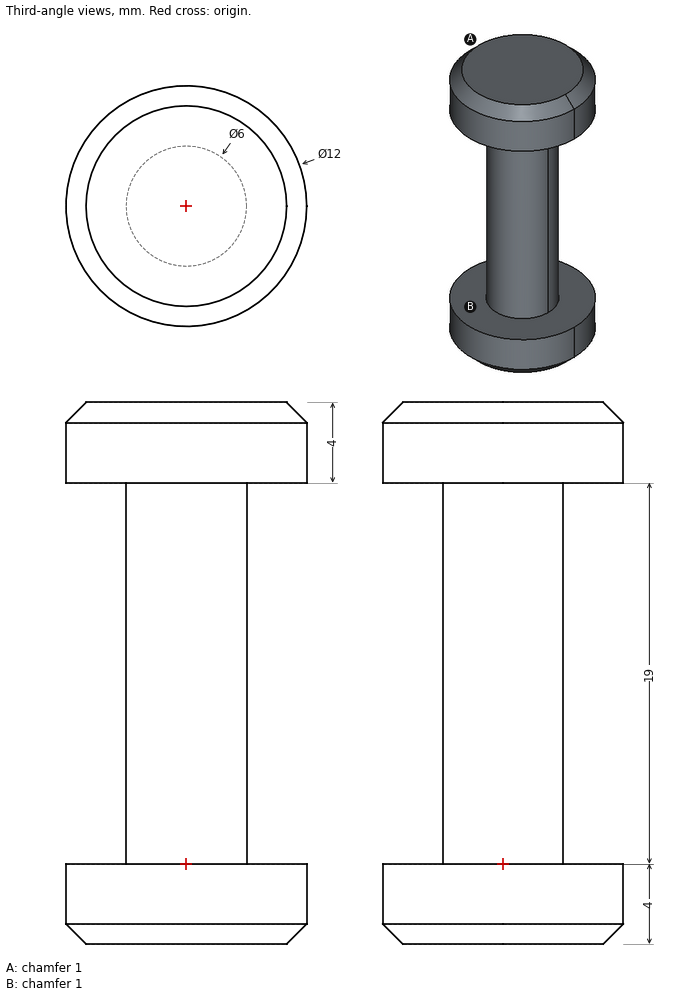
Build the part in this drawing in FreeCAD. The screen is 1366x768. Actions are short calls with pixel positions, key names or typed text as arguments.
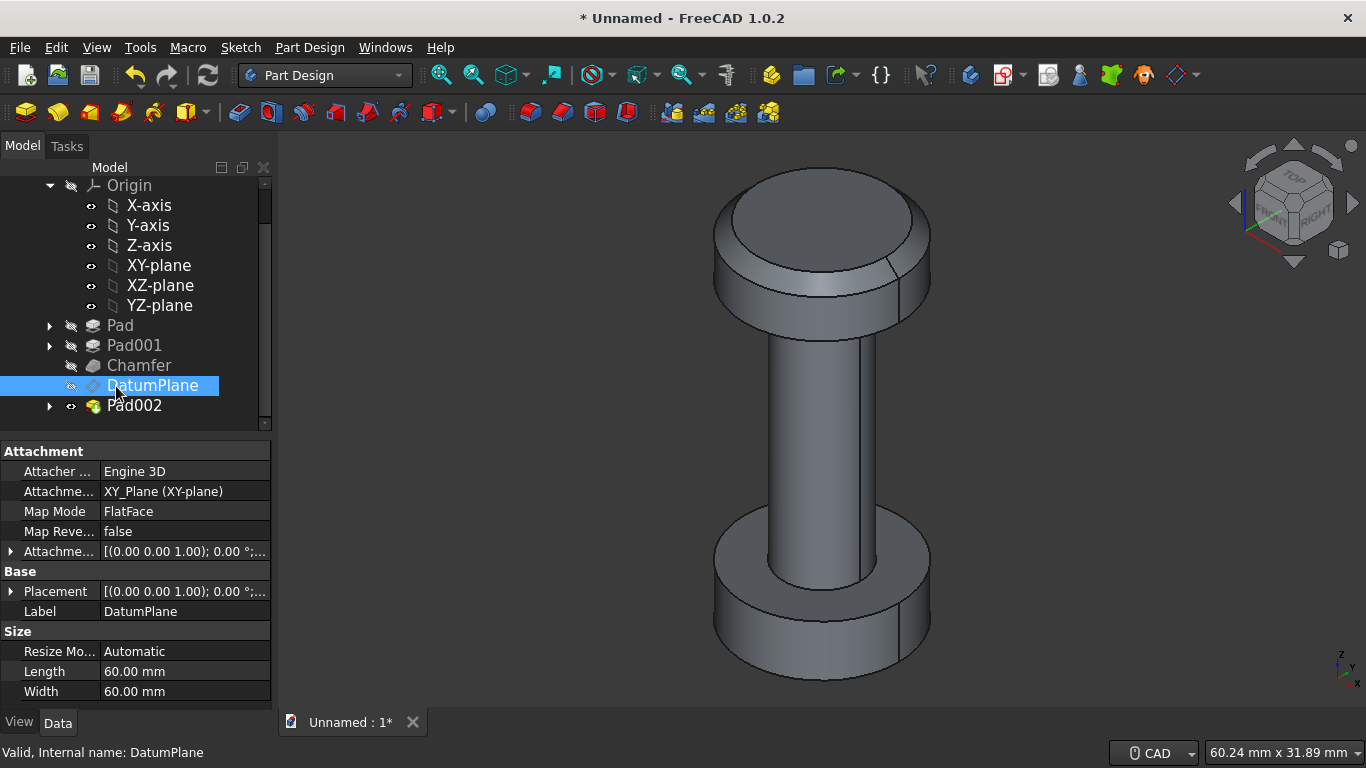
key(v)
key(f)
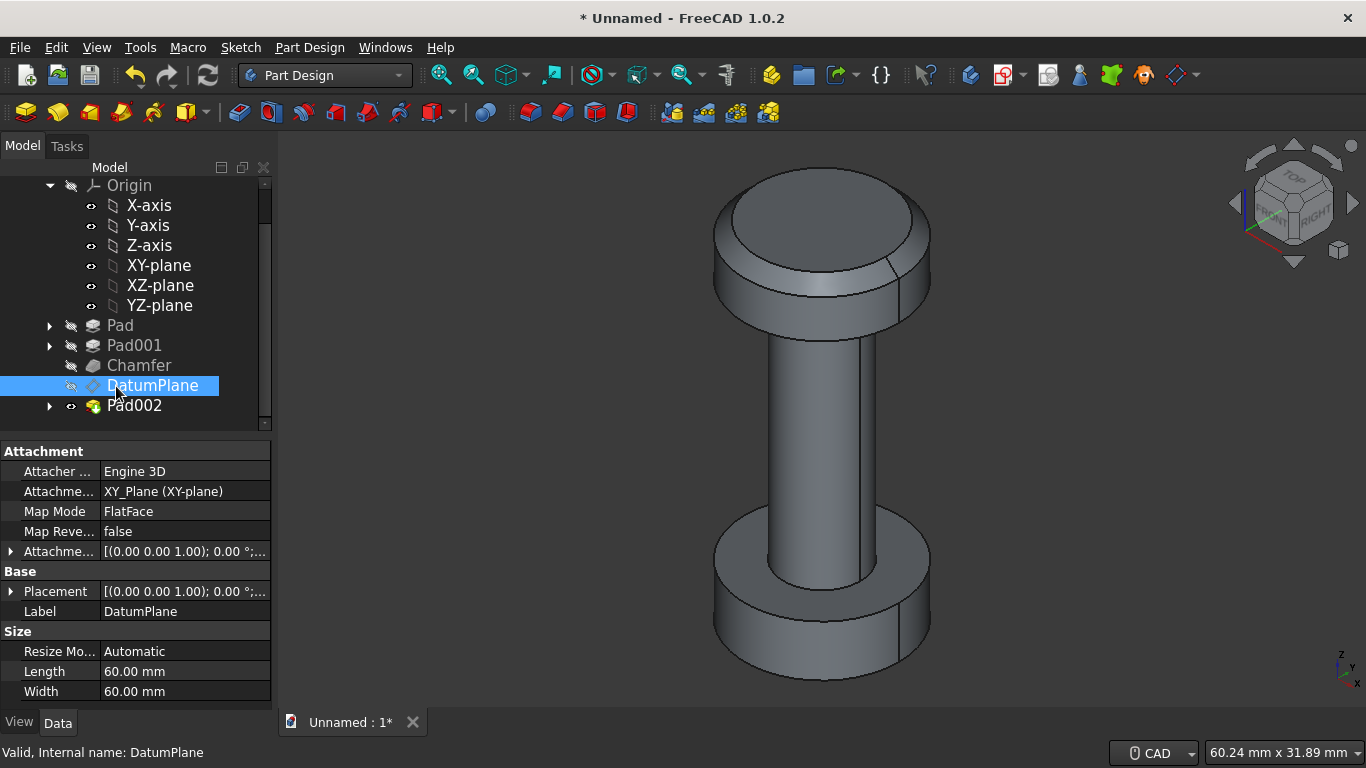
click(912, 652)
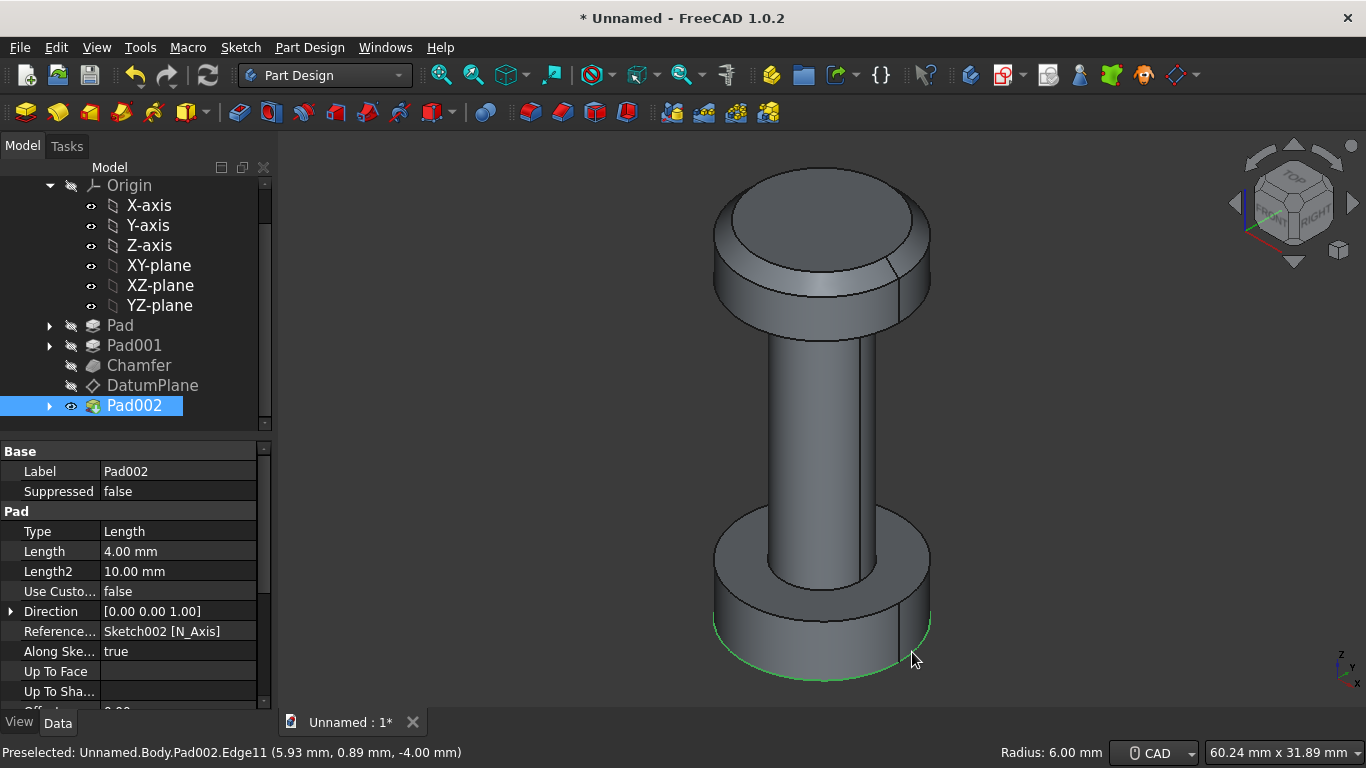
click(564, 112)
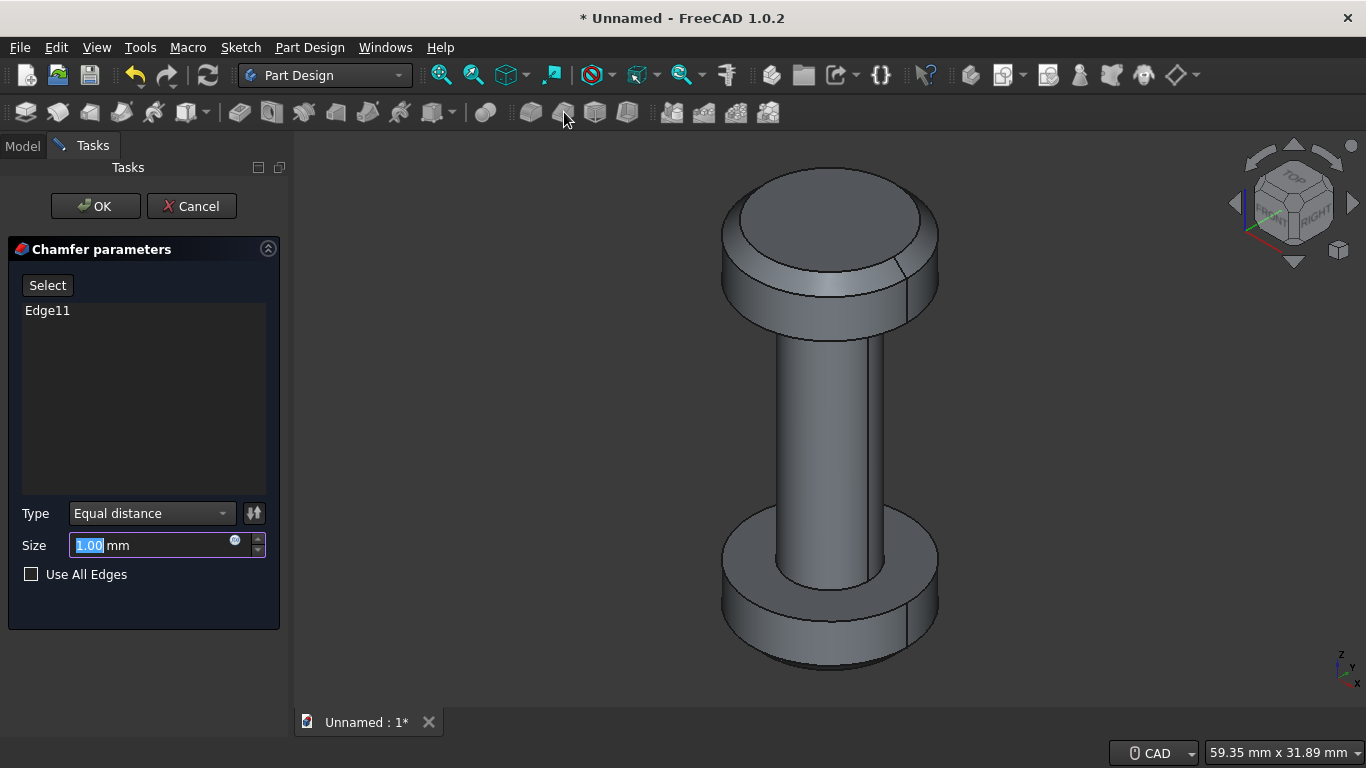
text(1)
key(Tab)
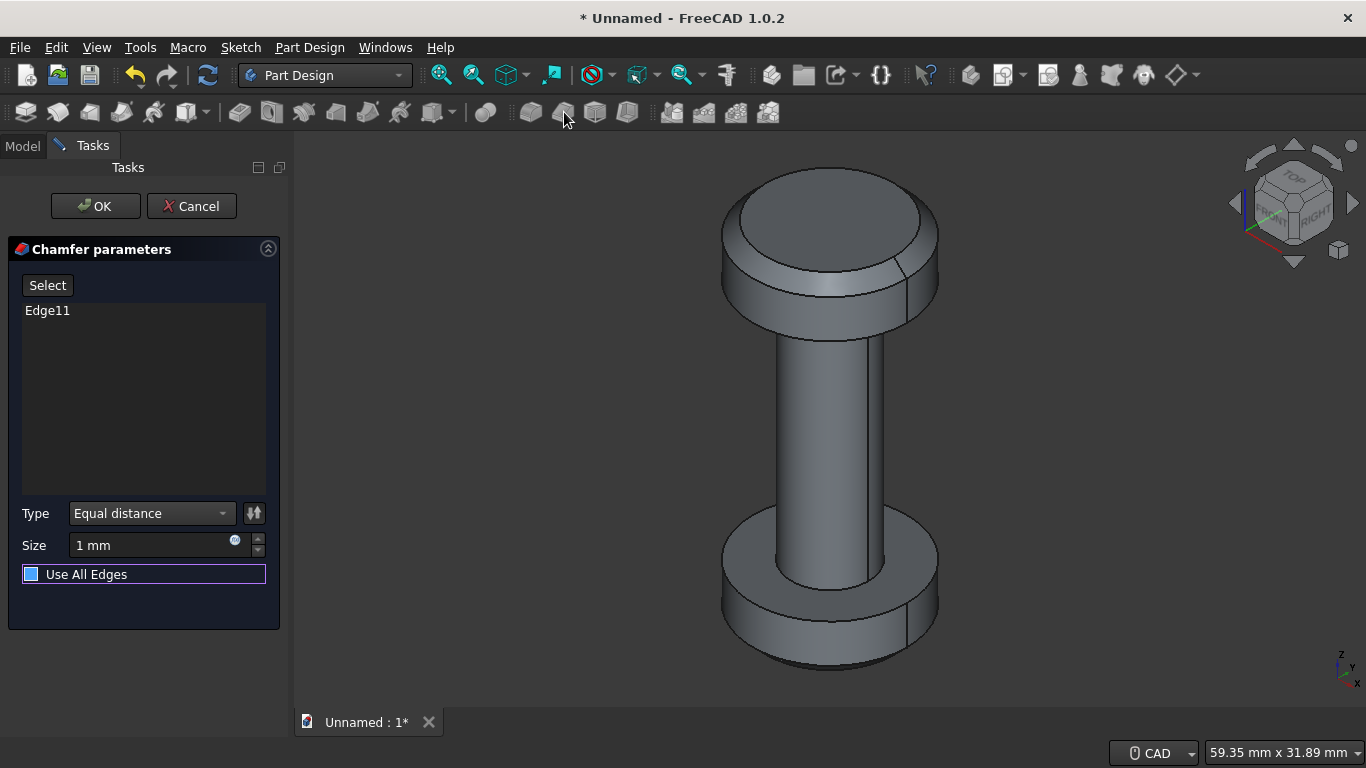
click(96, 206)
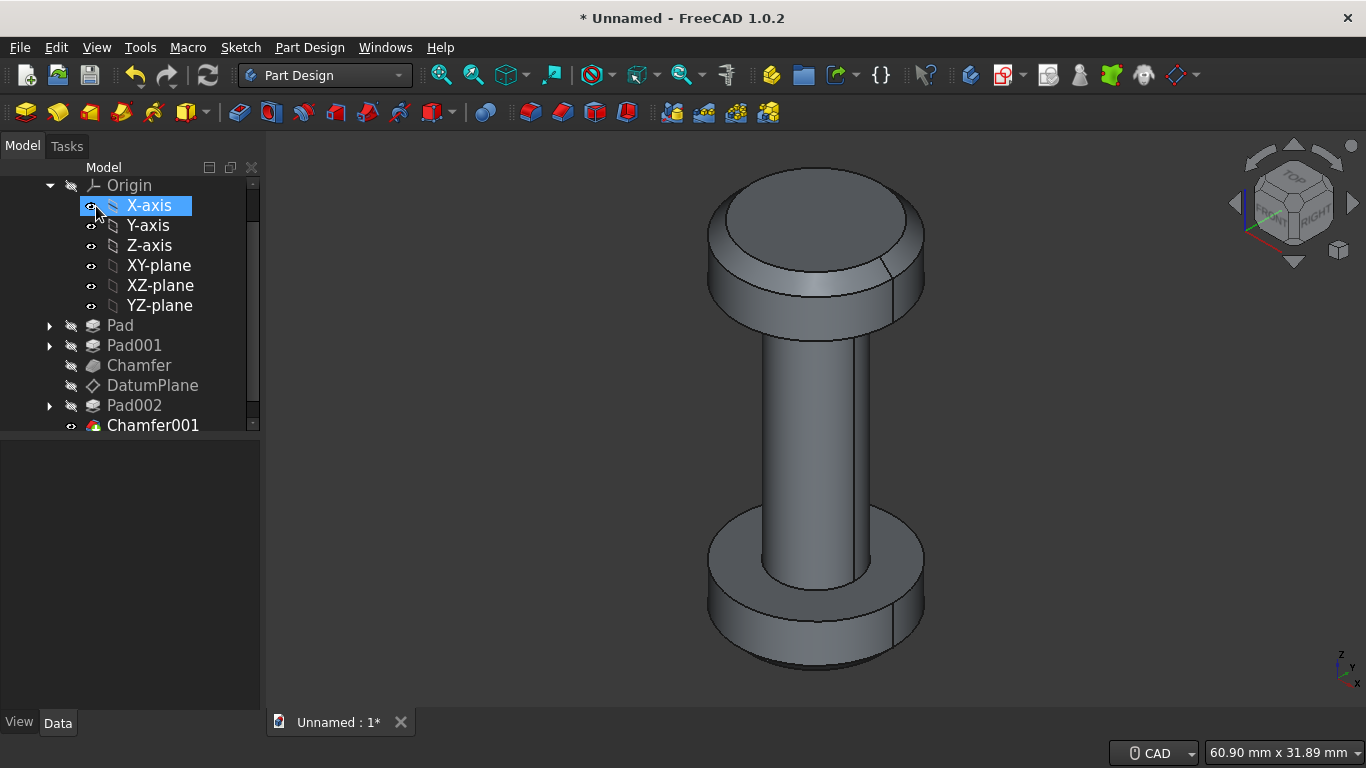
key(v)
key(f)